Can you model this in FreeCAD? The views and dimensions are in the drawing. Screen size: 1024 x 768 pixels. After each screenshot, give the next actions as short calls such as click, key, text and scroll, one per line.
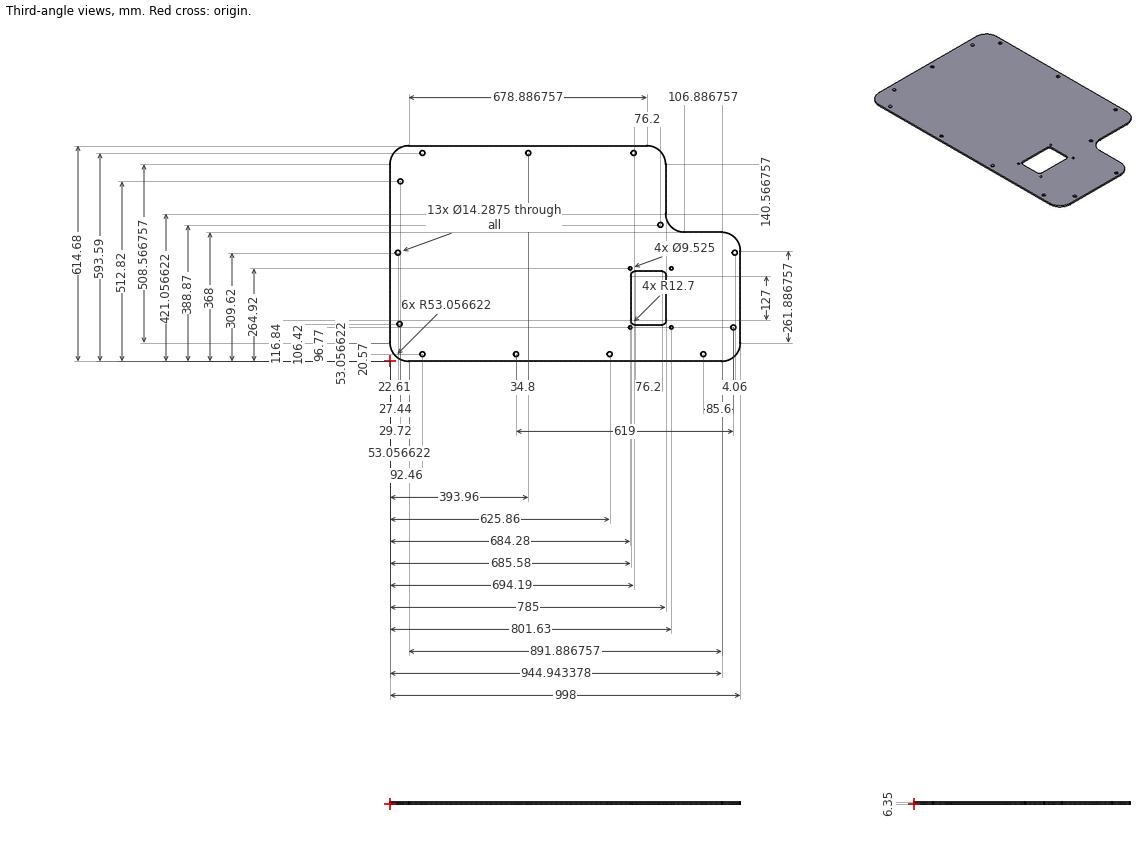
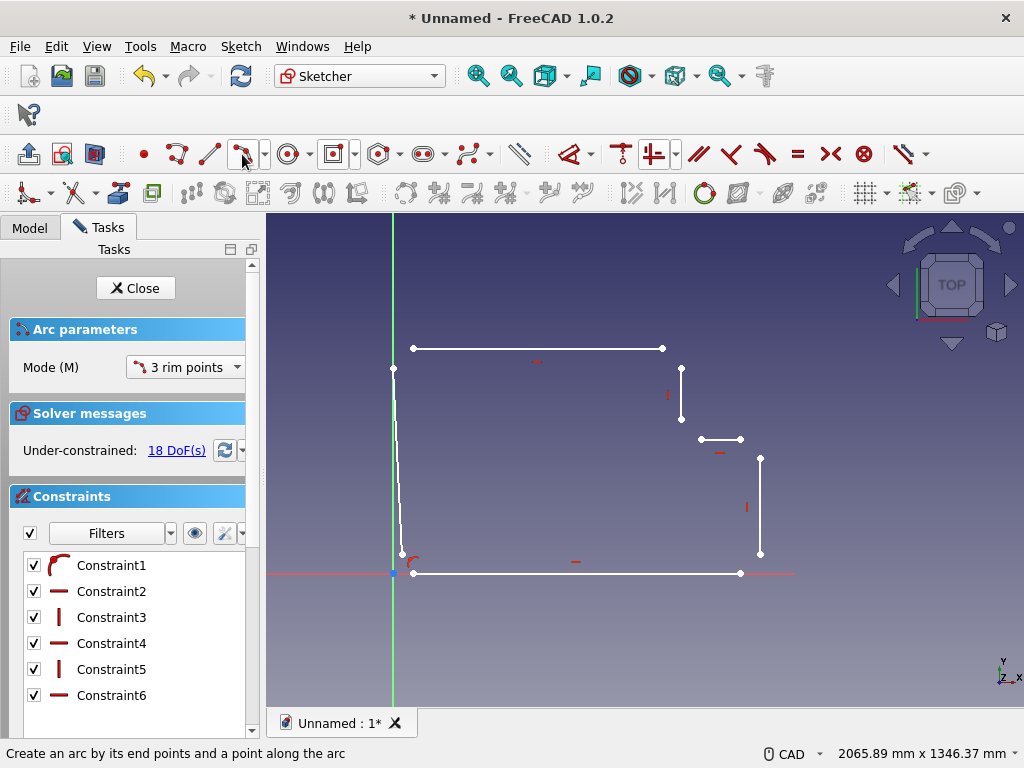
click(402, 555)
click(413, 574)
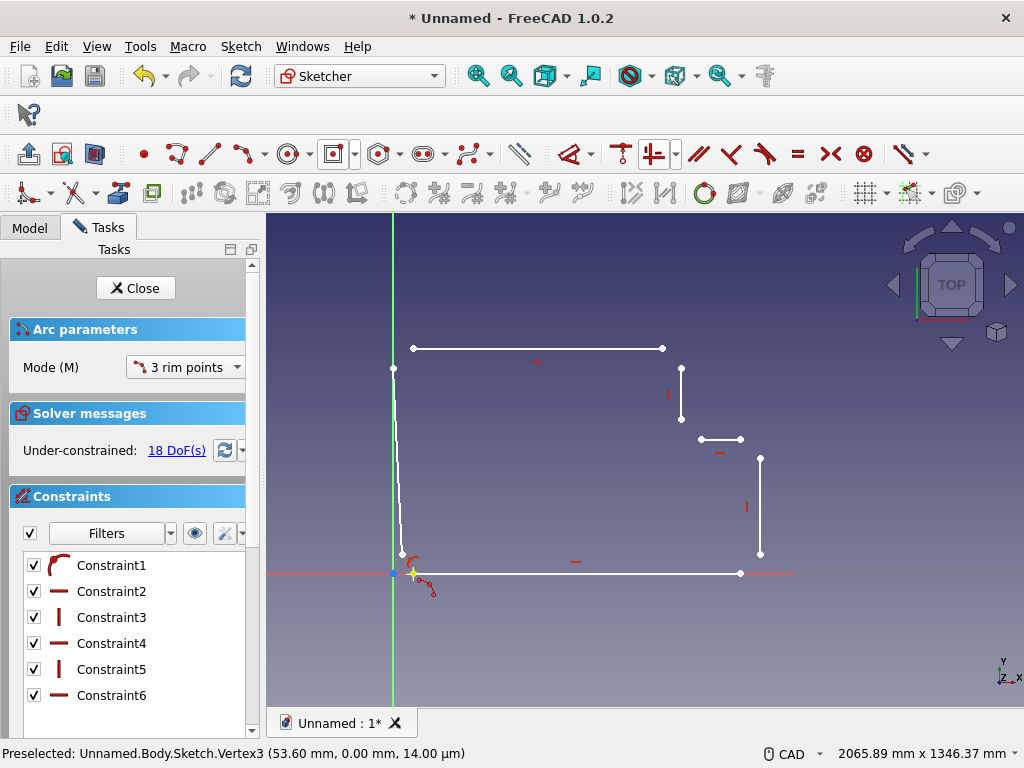
scroll(399, 568, up, 6)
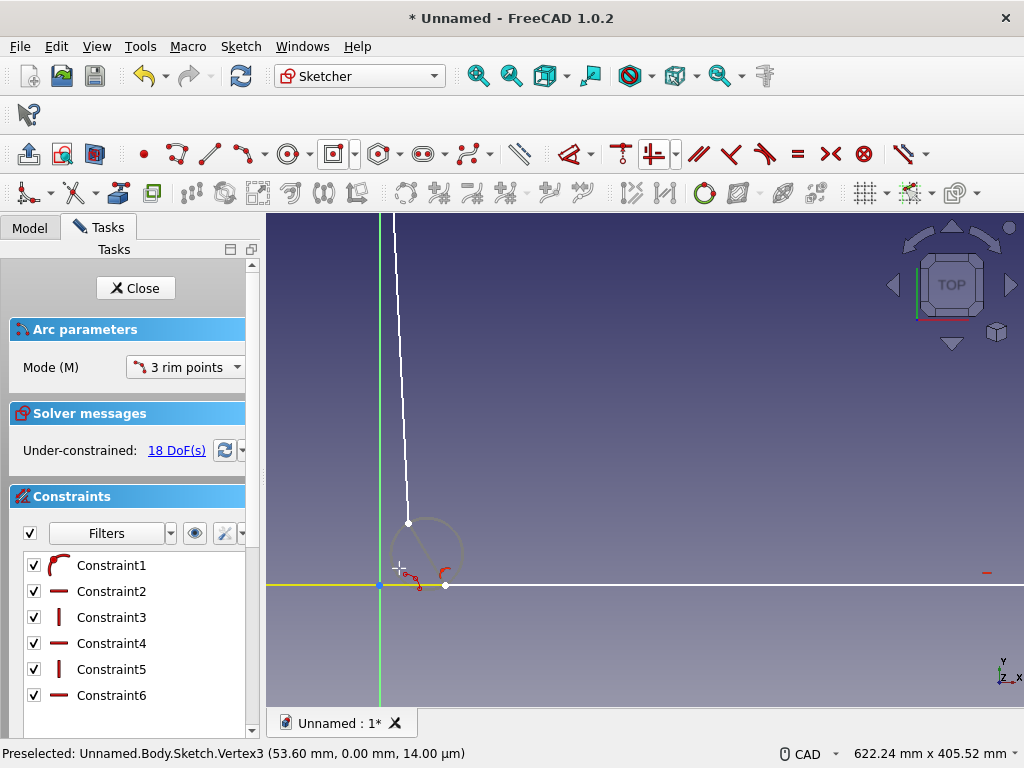
click(399, 566)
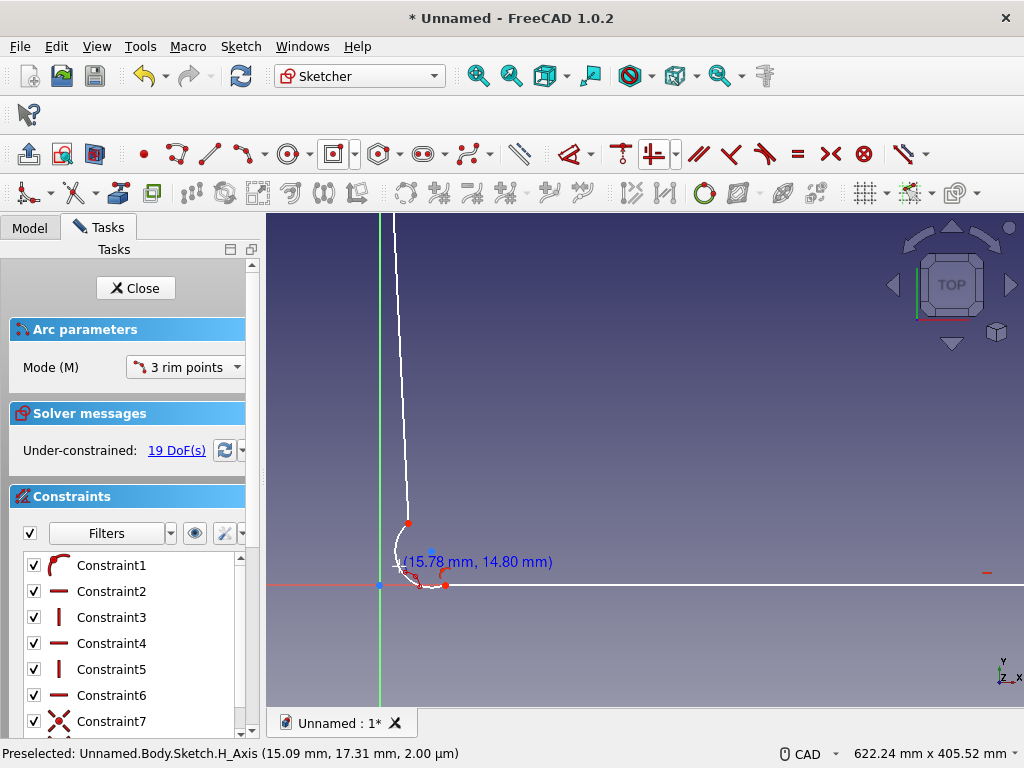
scroll(399, 567, down, 6)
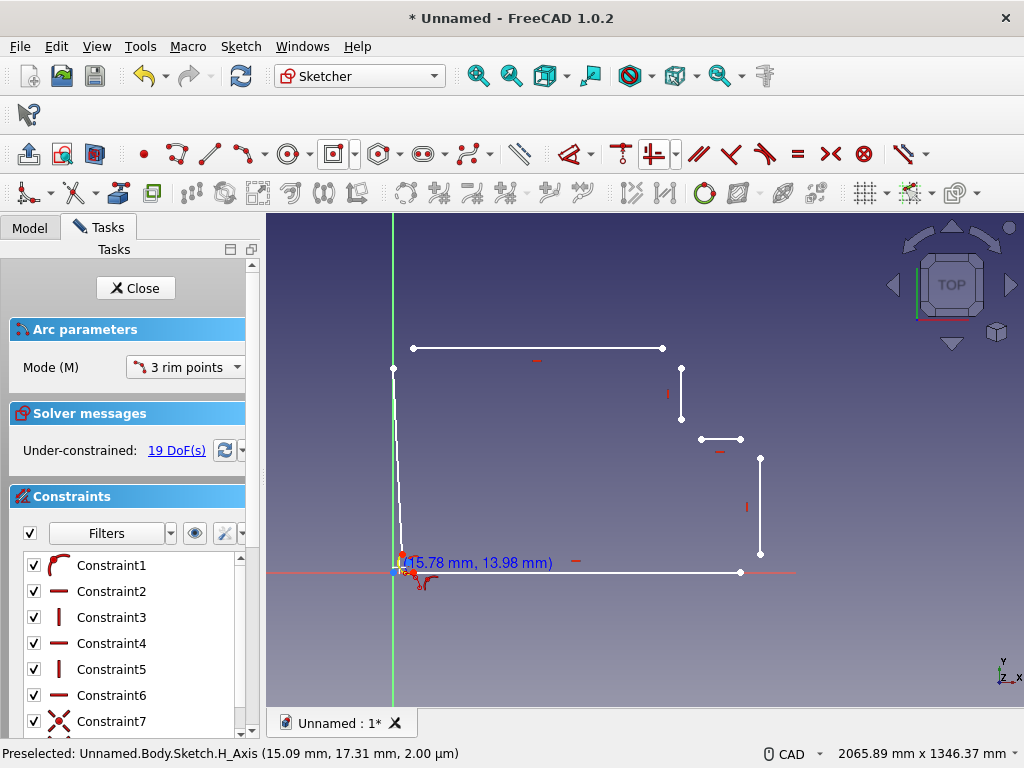
click(740, 573)
click(760, 554)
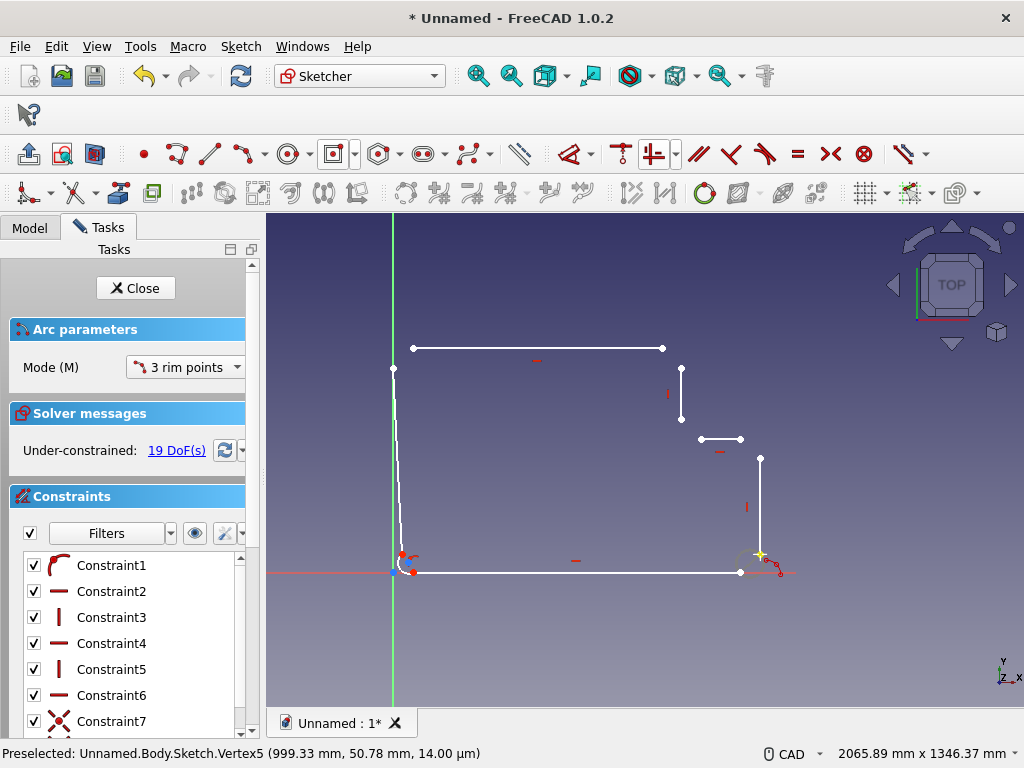
scroll(754, 567, up, 6)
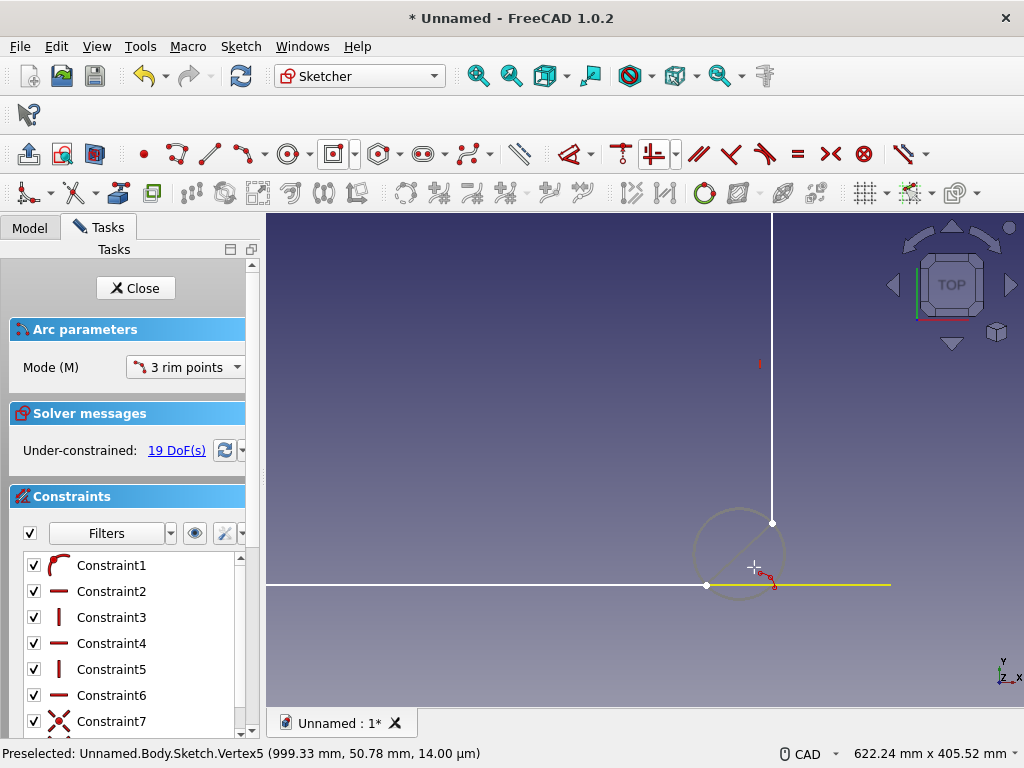
click(752, 566)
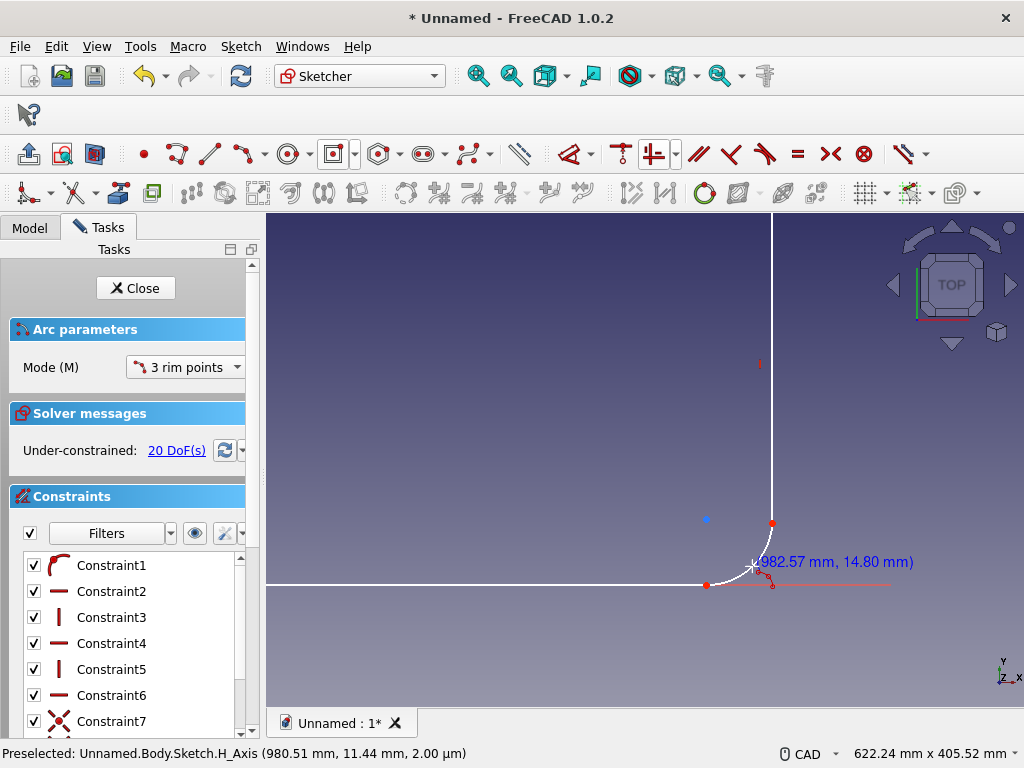
scroll(755, 567, down, 6)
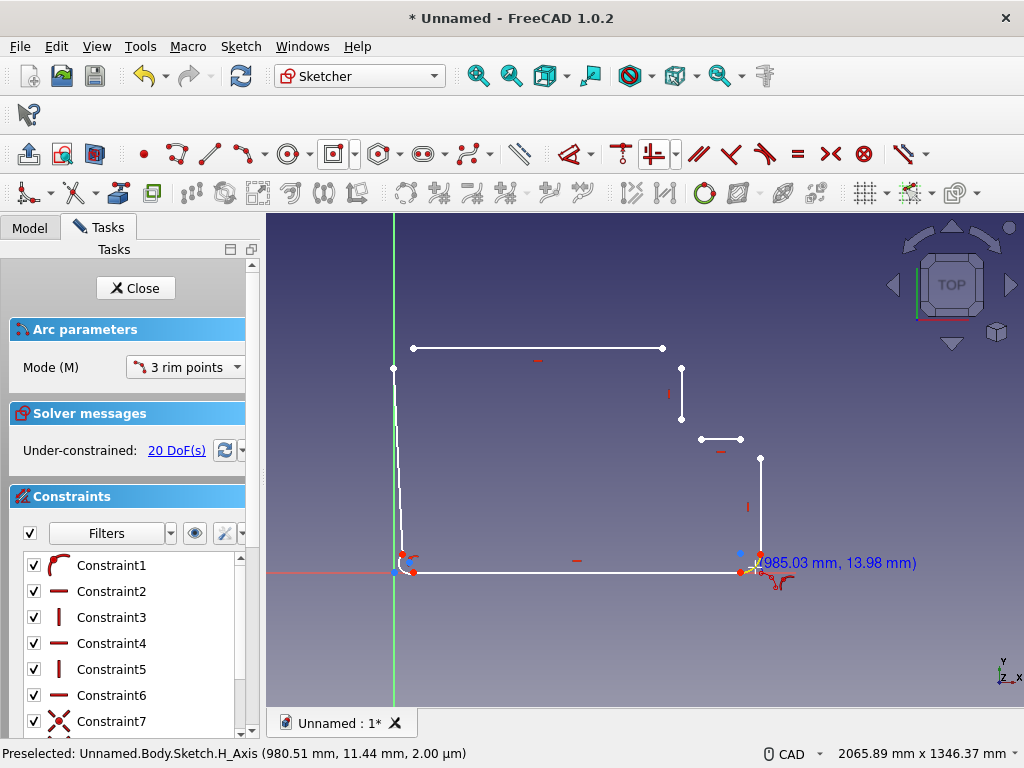
click(761, 458)
click(741, 439)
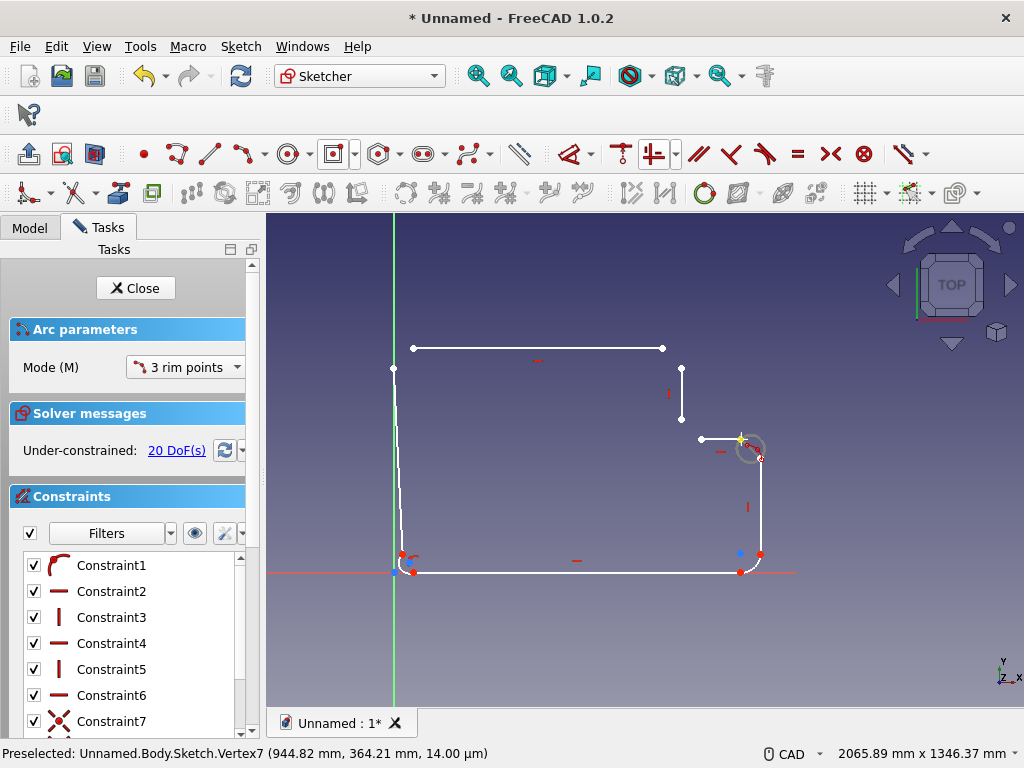
scroll(755, 444, up, 6)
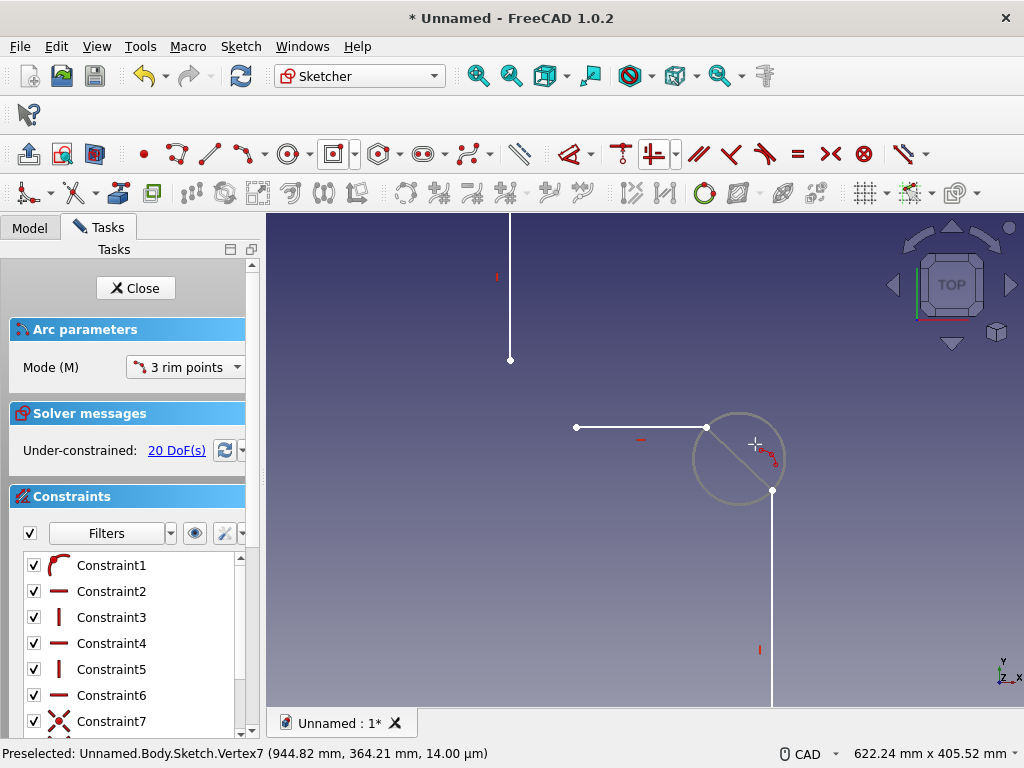
click(752, 442)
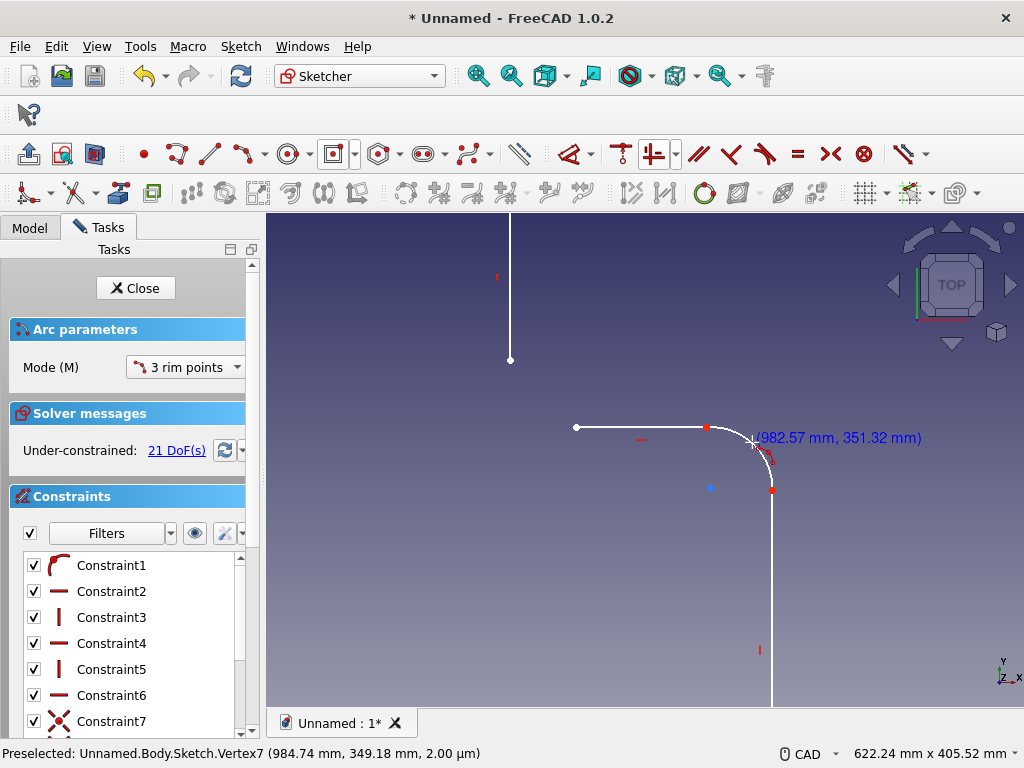
click(577, 427)
click(510, 361)
click(530, 404)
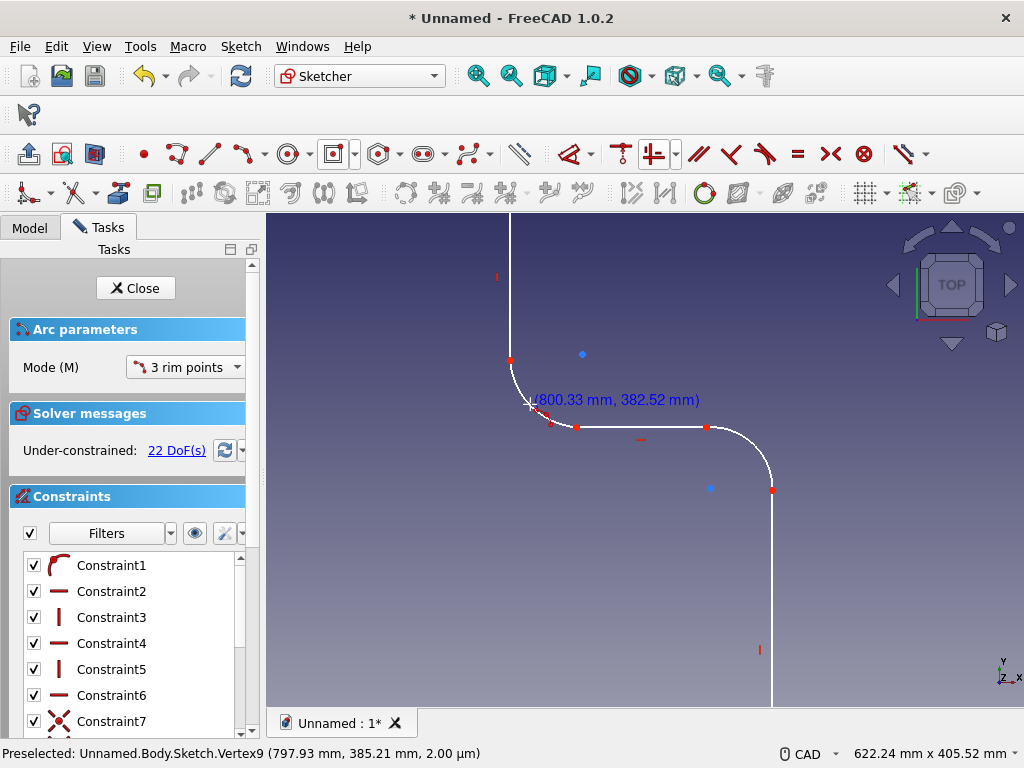
scroll(755, 444, down, 6)